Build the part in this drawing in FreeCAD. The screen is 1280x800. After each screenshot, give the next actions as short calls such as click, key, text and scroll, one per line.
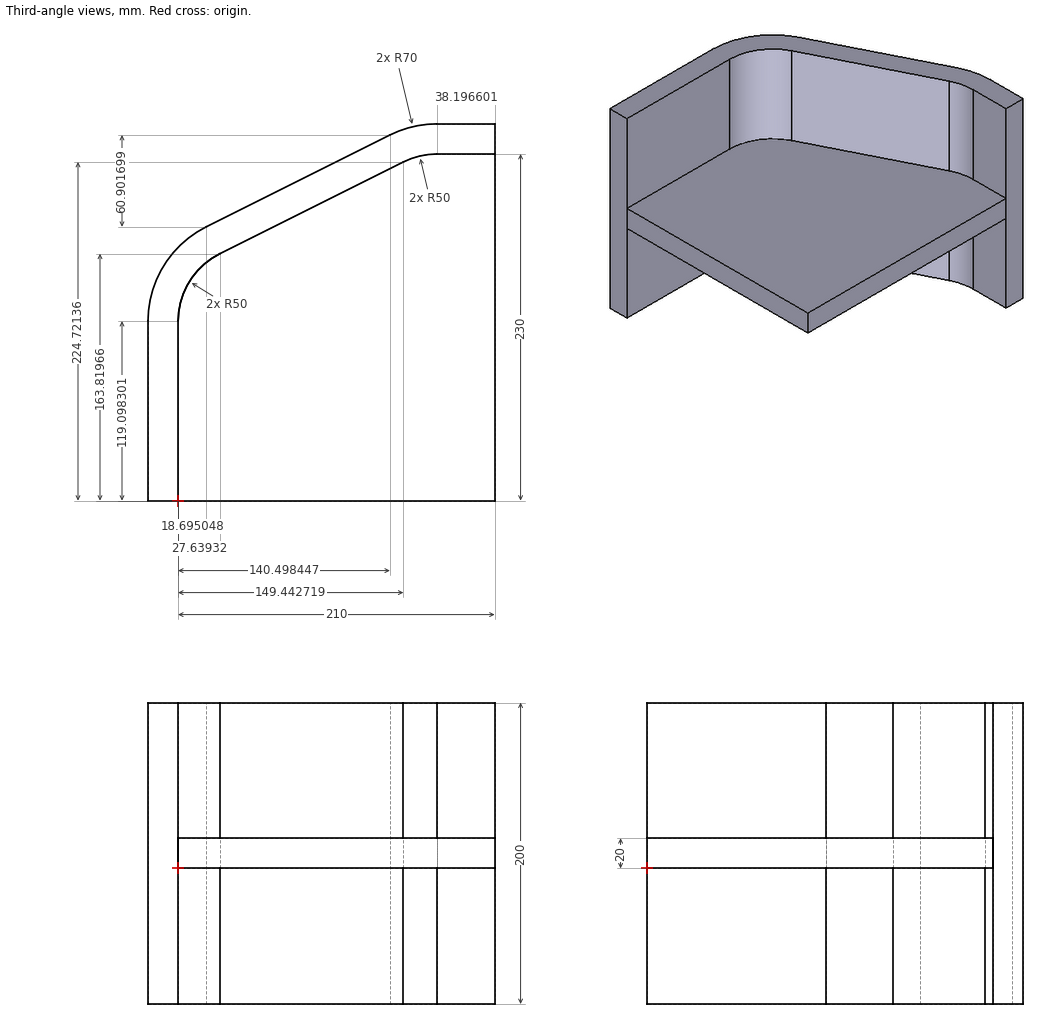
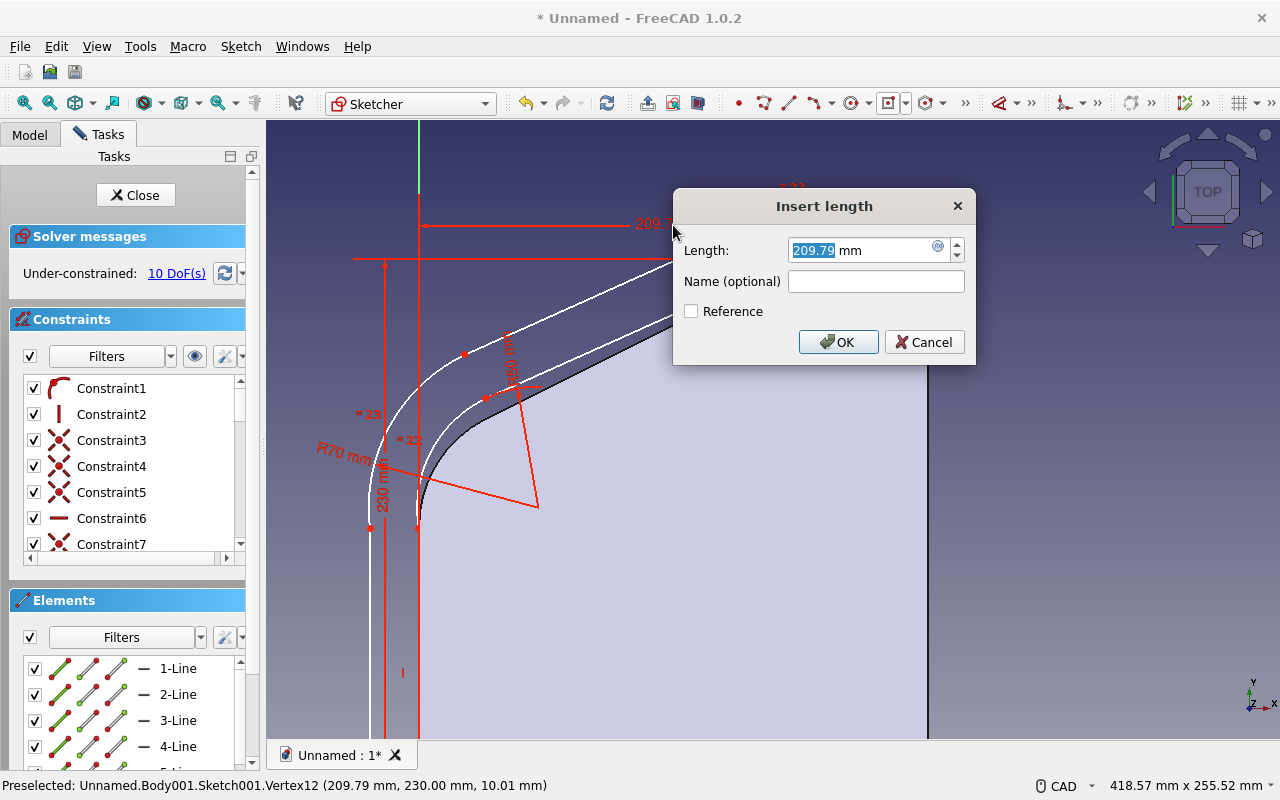
text(210)
key(Return)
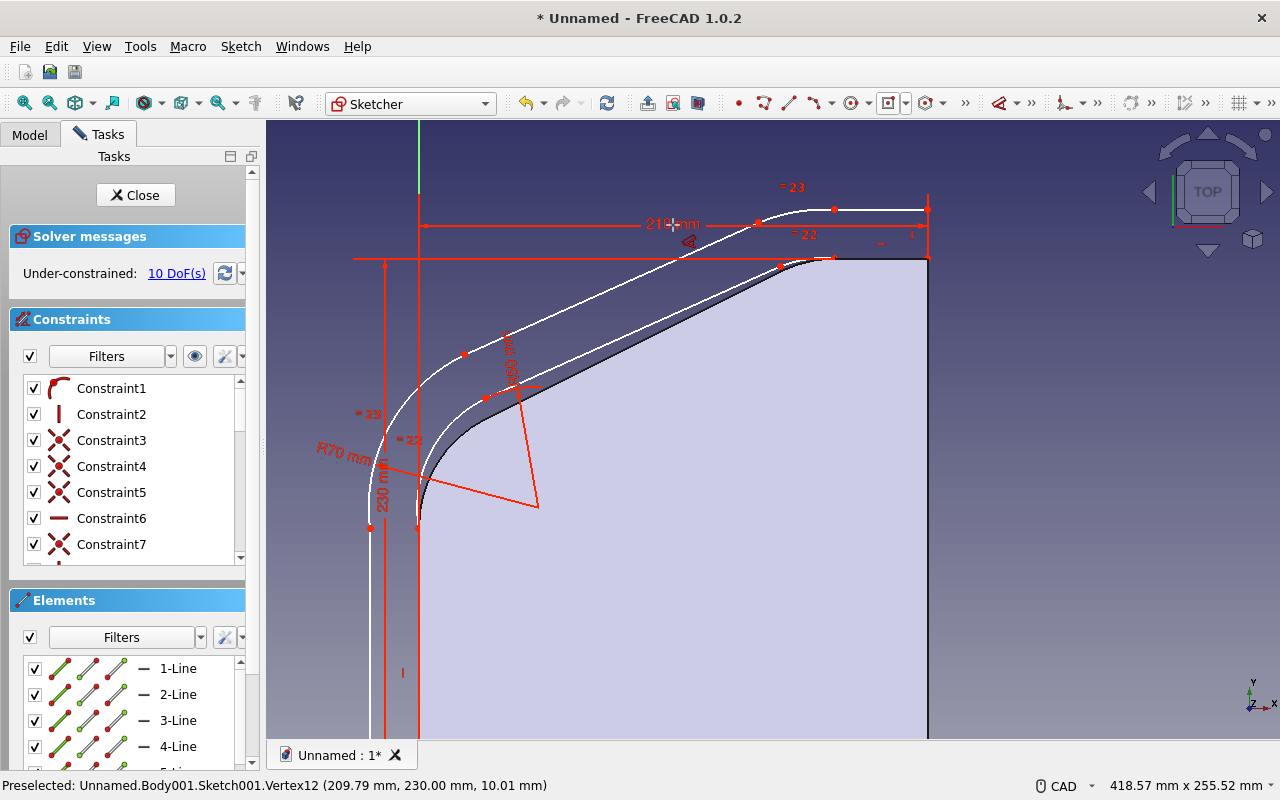
click(863, 259)
click(881, 225)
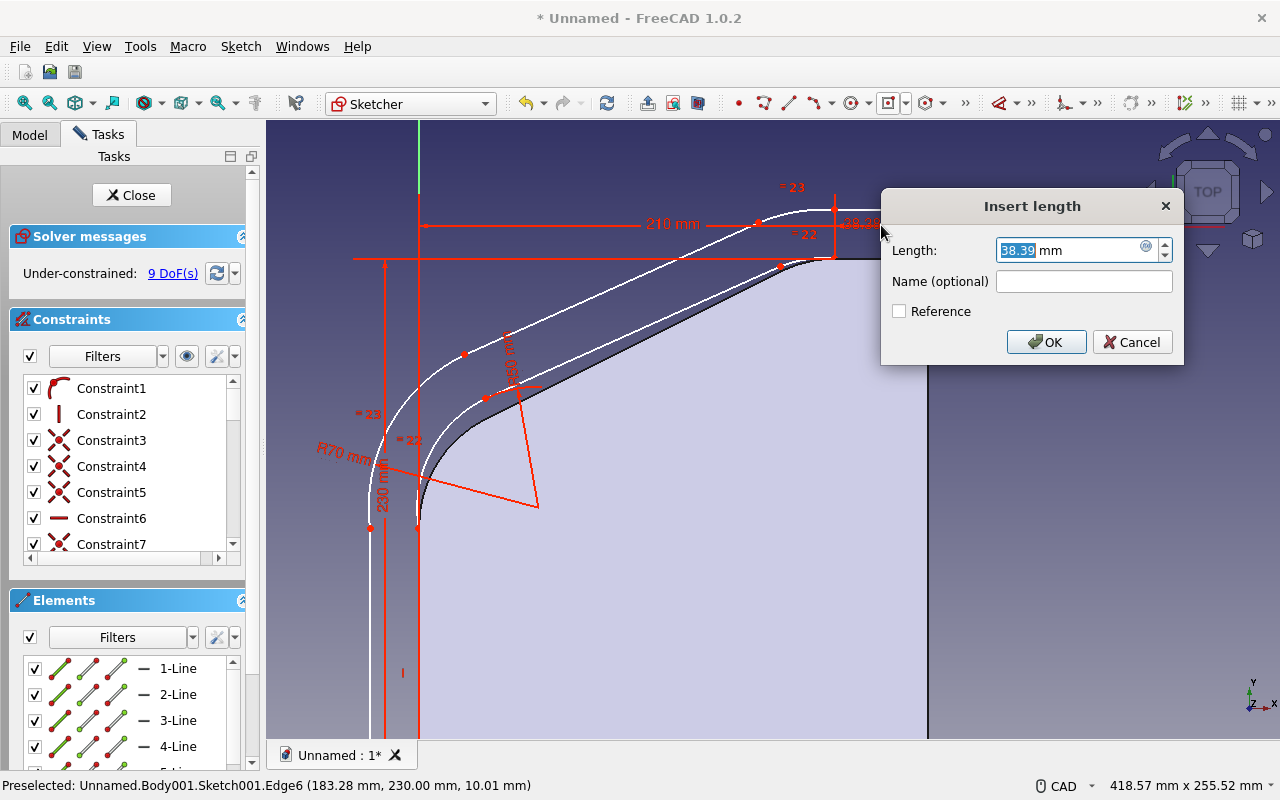
text(38.196601)
key(Return)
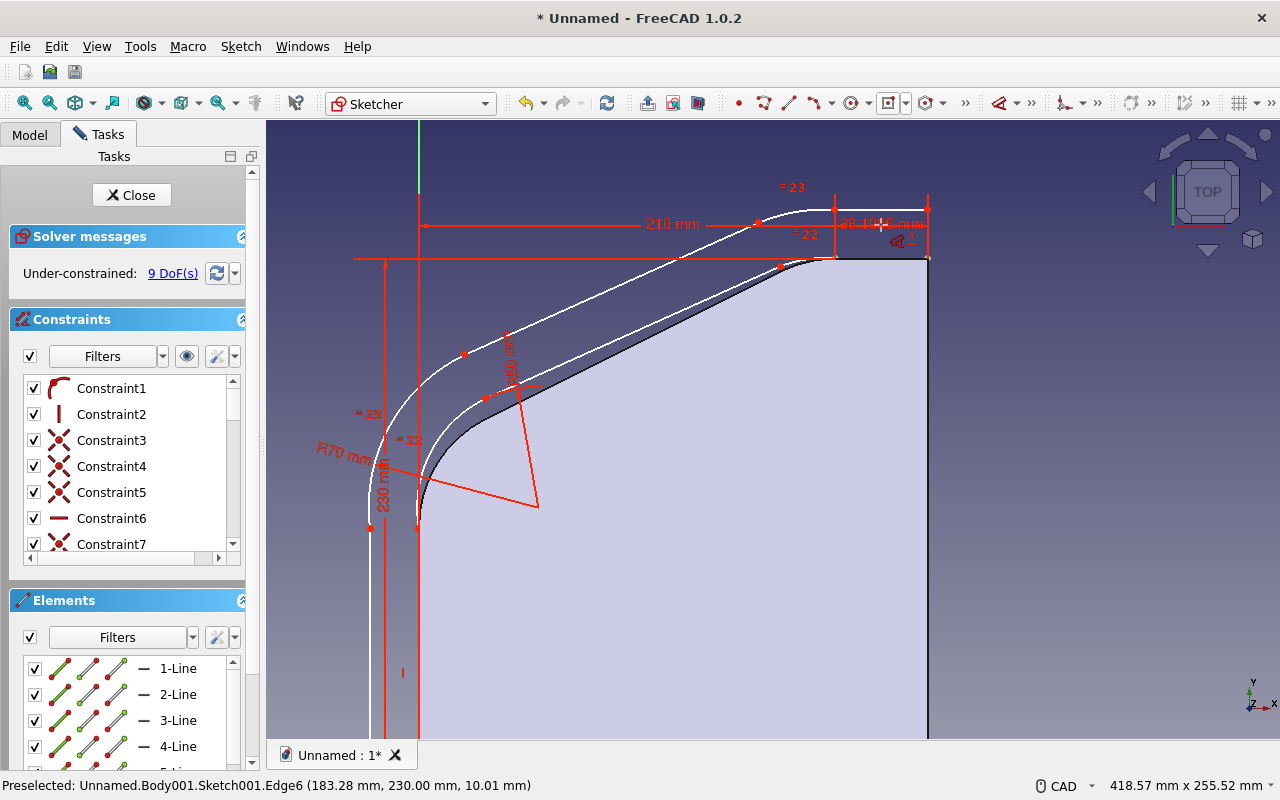
click(900, 210)
click(881, 176)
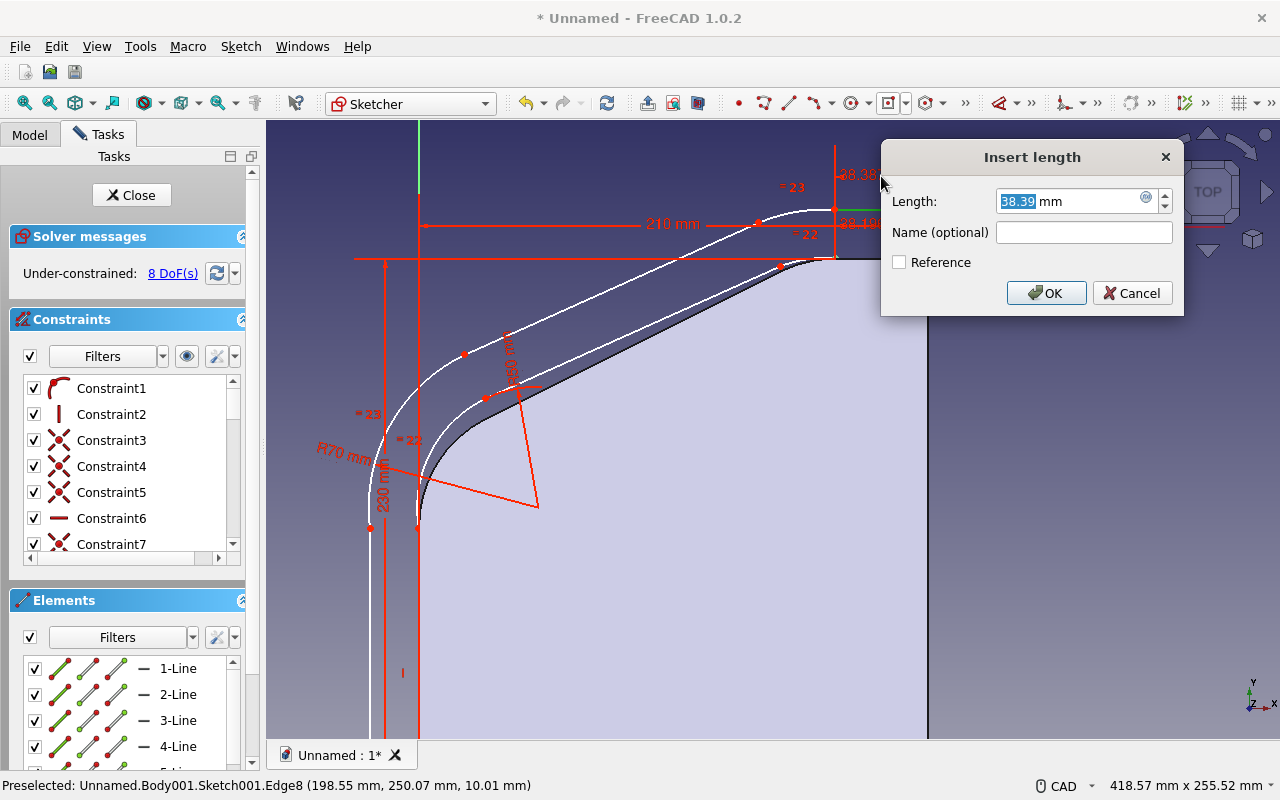
text(38.196601)
key(Return)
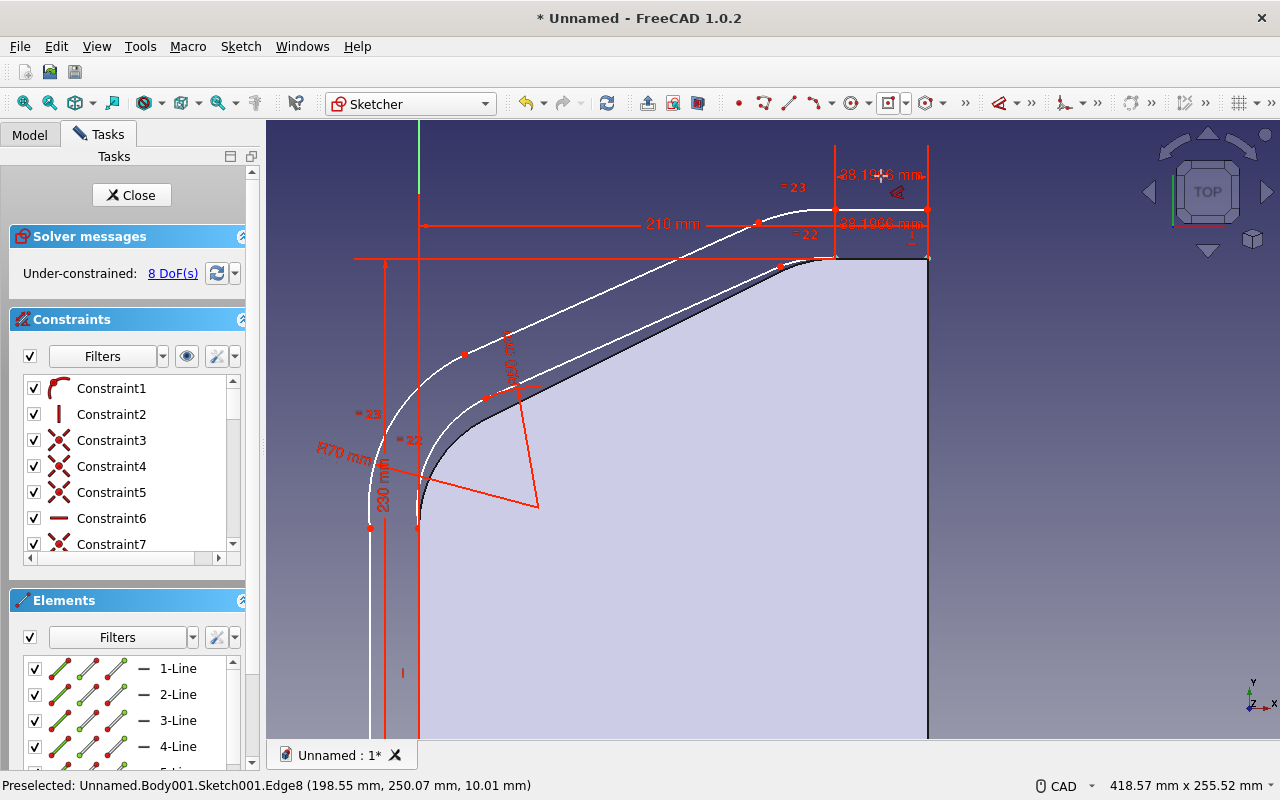
click(486, 399)
click(476, 365)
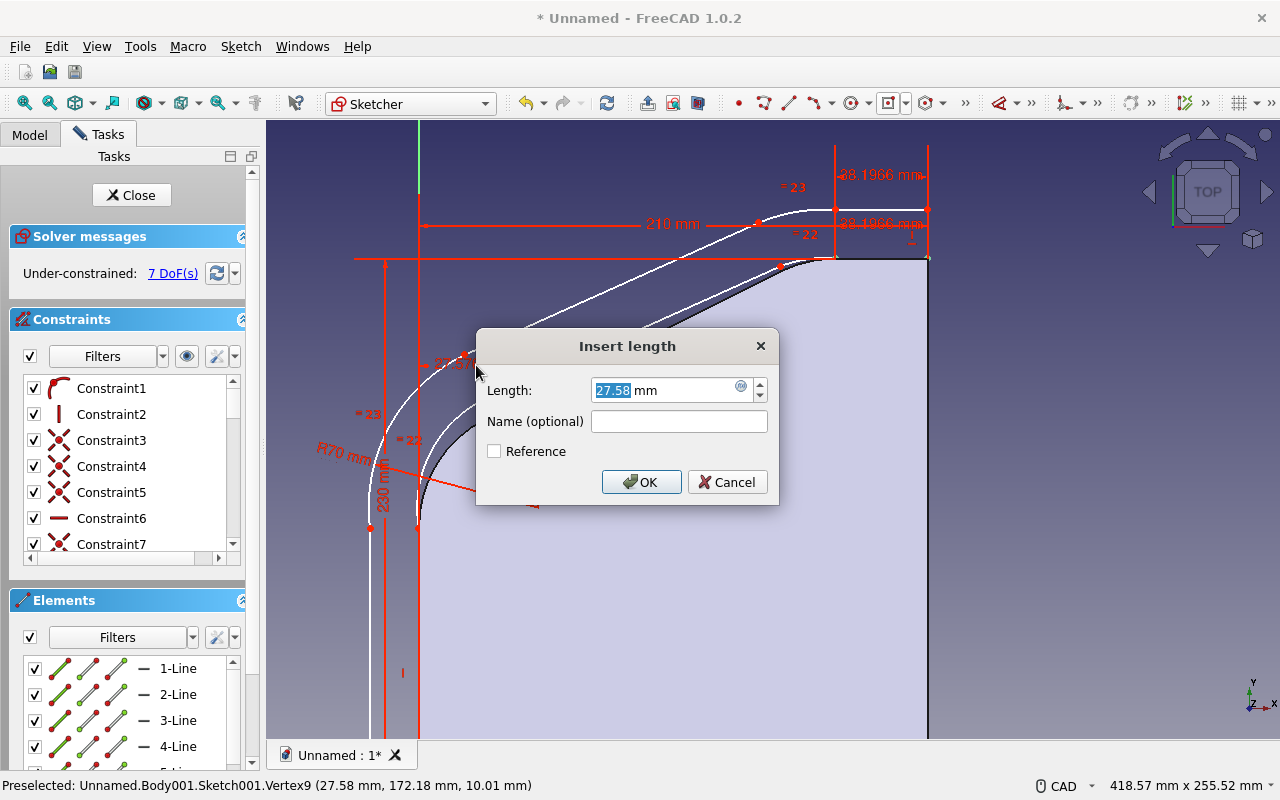
text(27.63932)
key(Return)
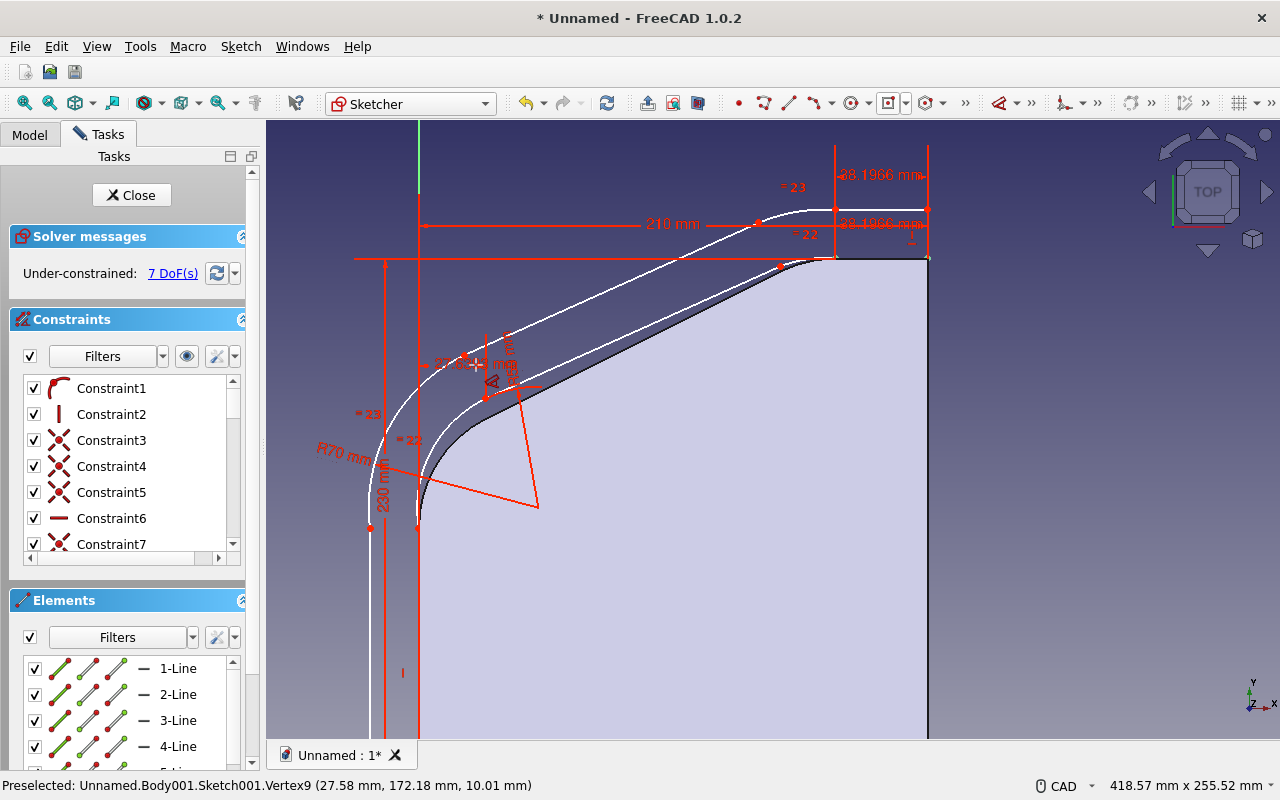
click(370, 615)
click(336, 620)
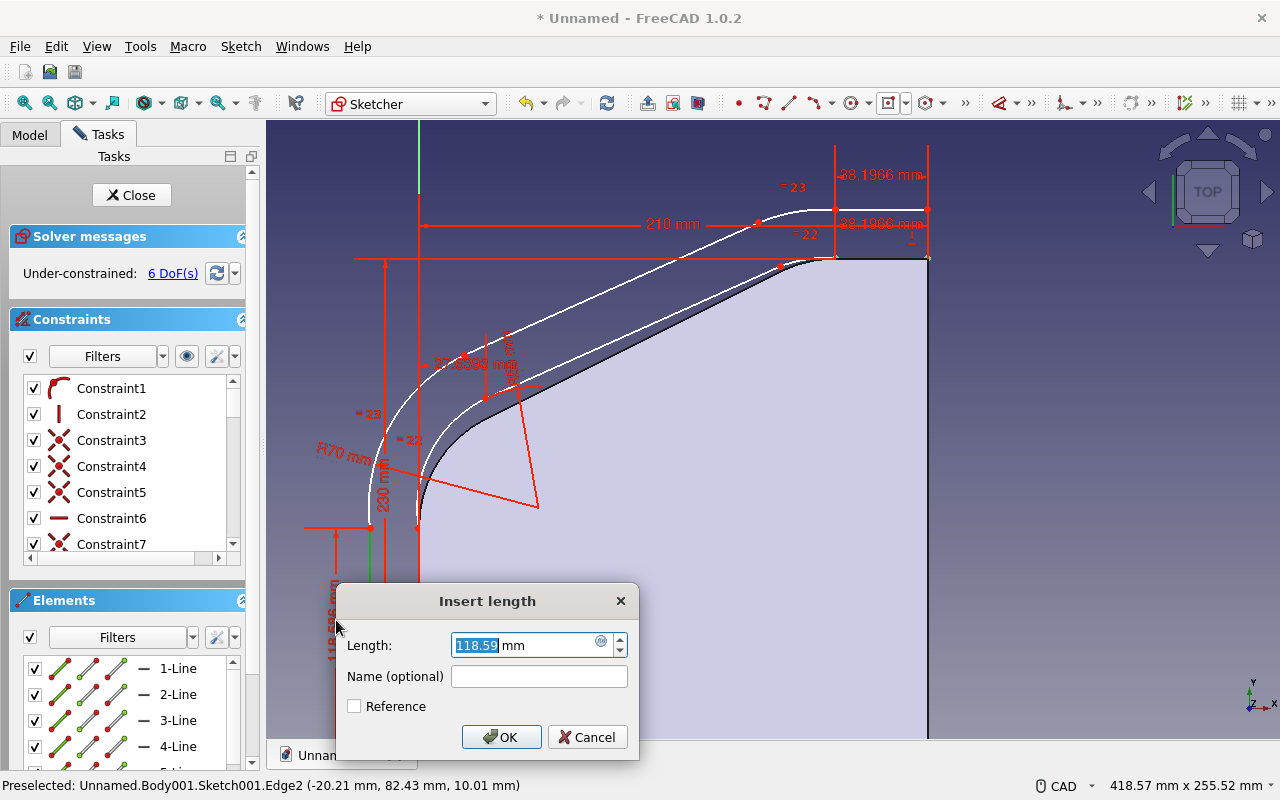
text(119.098301)
key(Return)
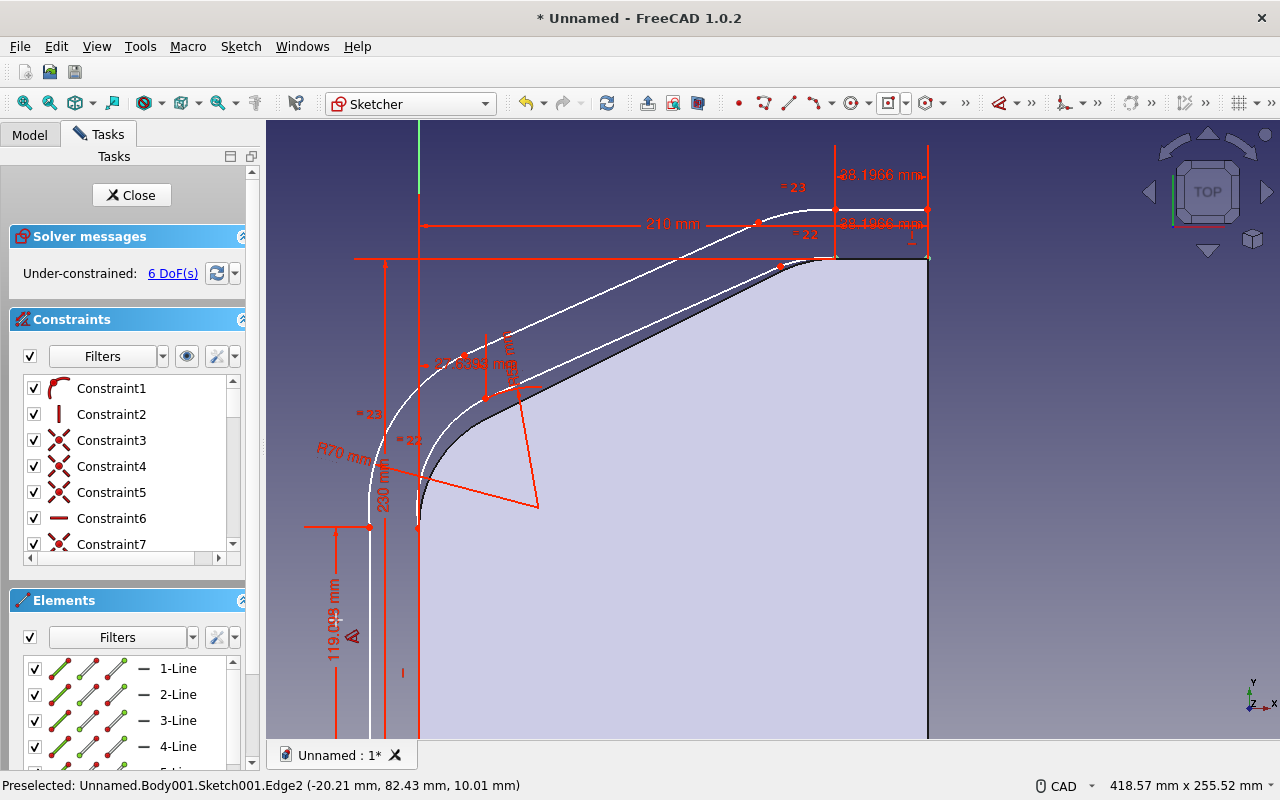
click(419, 615)
click(385, 578)